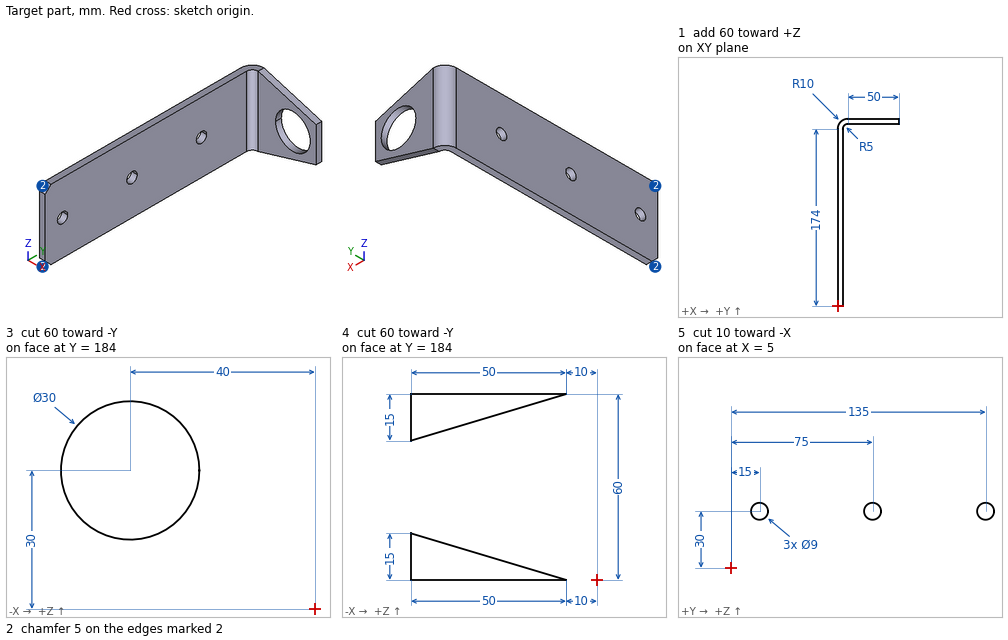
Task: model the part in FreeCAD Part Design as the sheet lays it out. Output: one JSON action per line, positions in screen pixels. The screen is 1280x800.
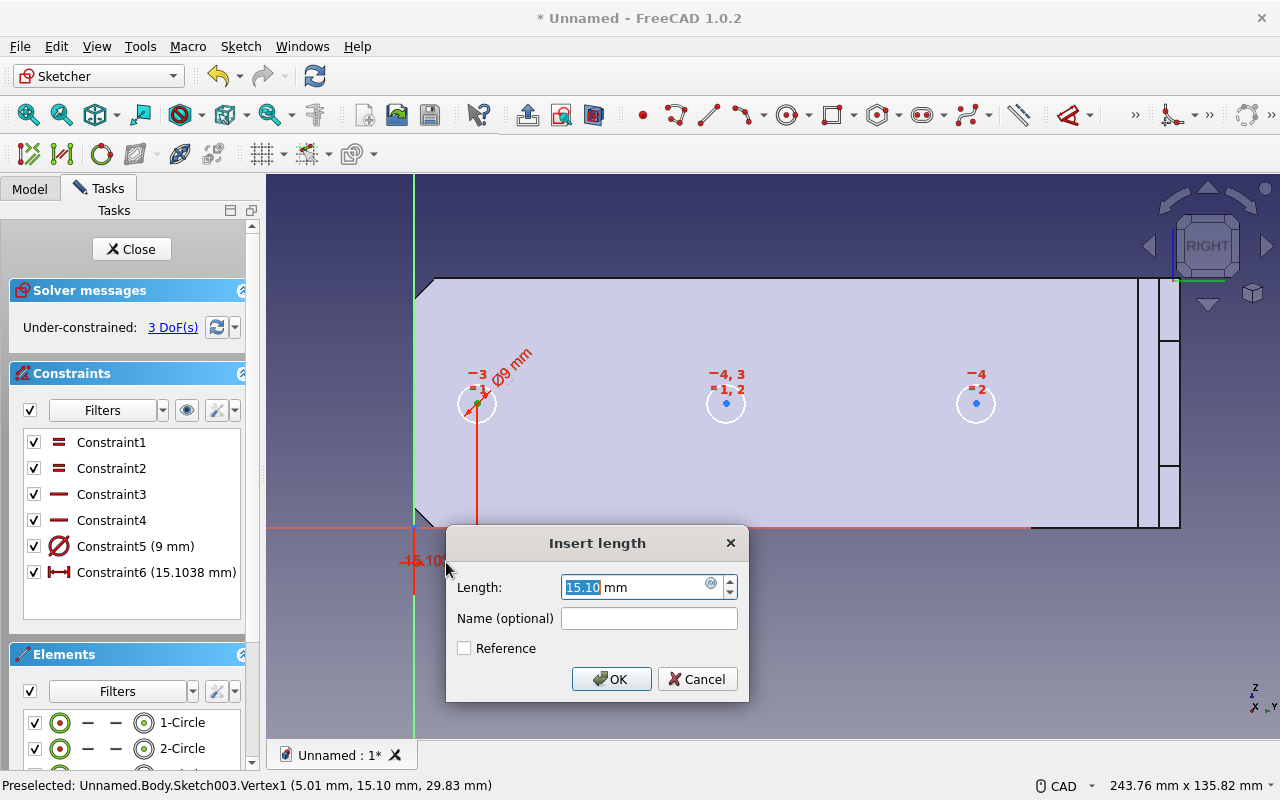
{"action": "type", "text": "15"}
{"action": "key", "text": "Return"}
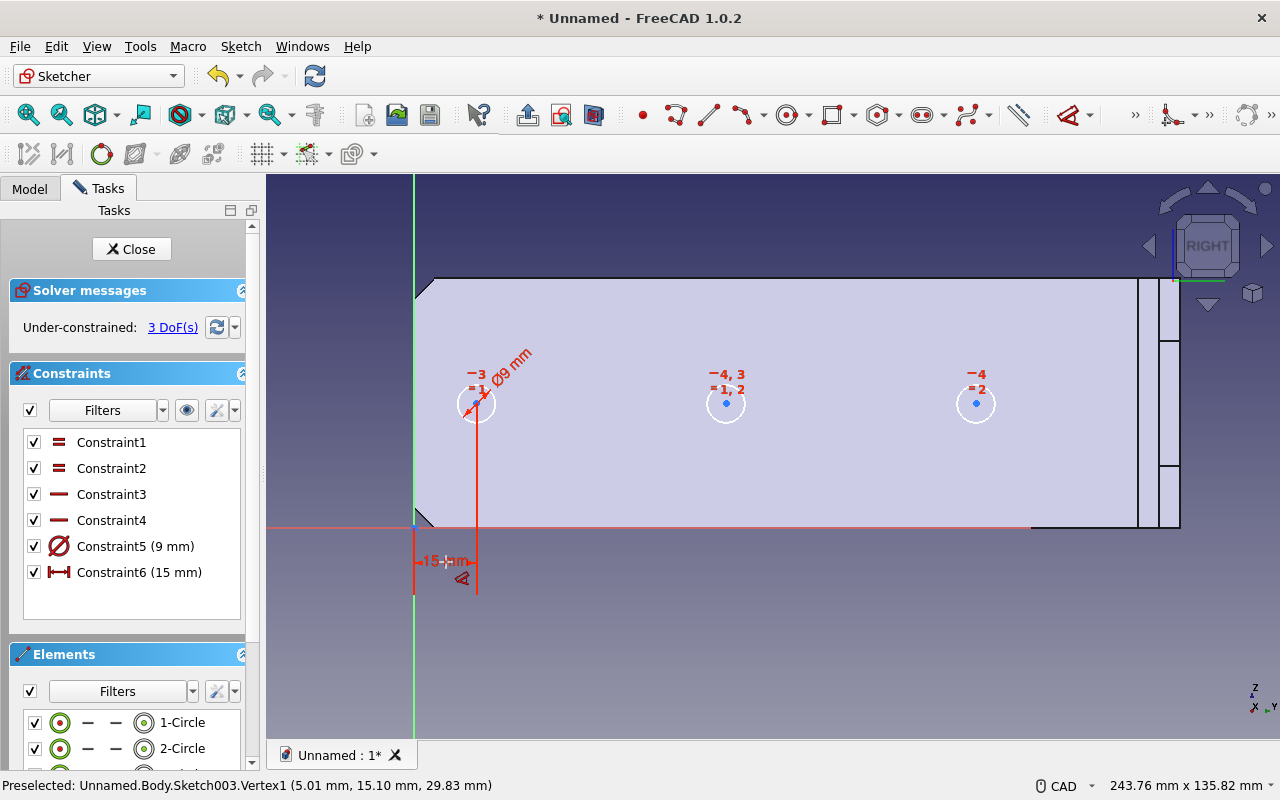
{"action": "left_click", "coordinate": [477, 404]}
{"action": "left_click", "coordinate": [380, 466]}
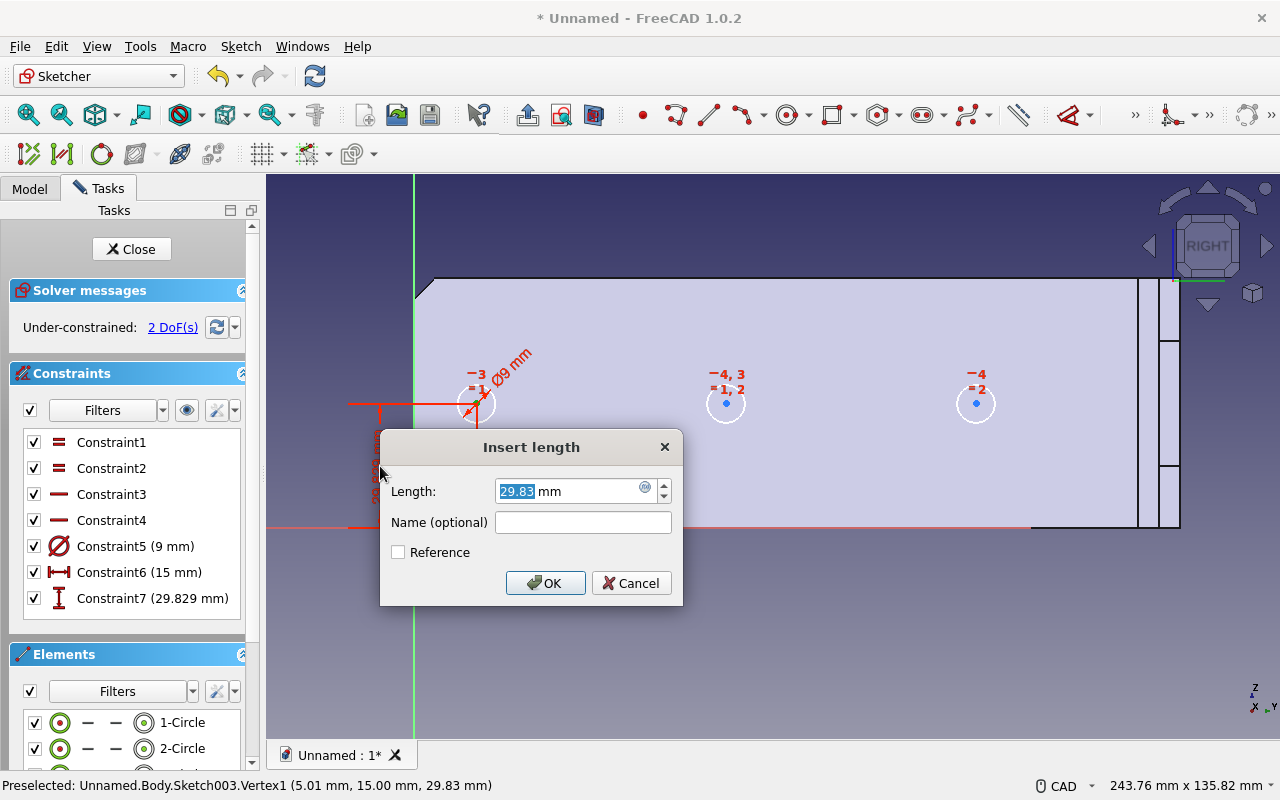
{"action": "type", "text": "30"}
{"action": "key", "text": "Return"}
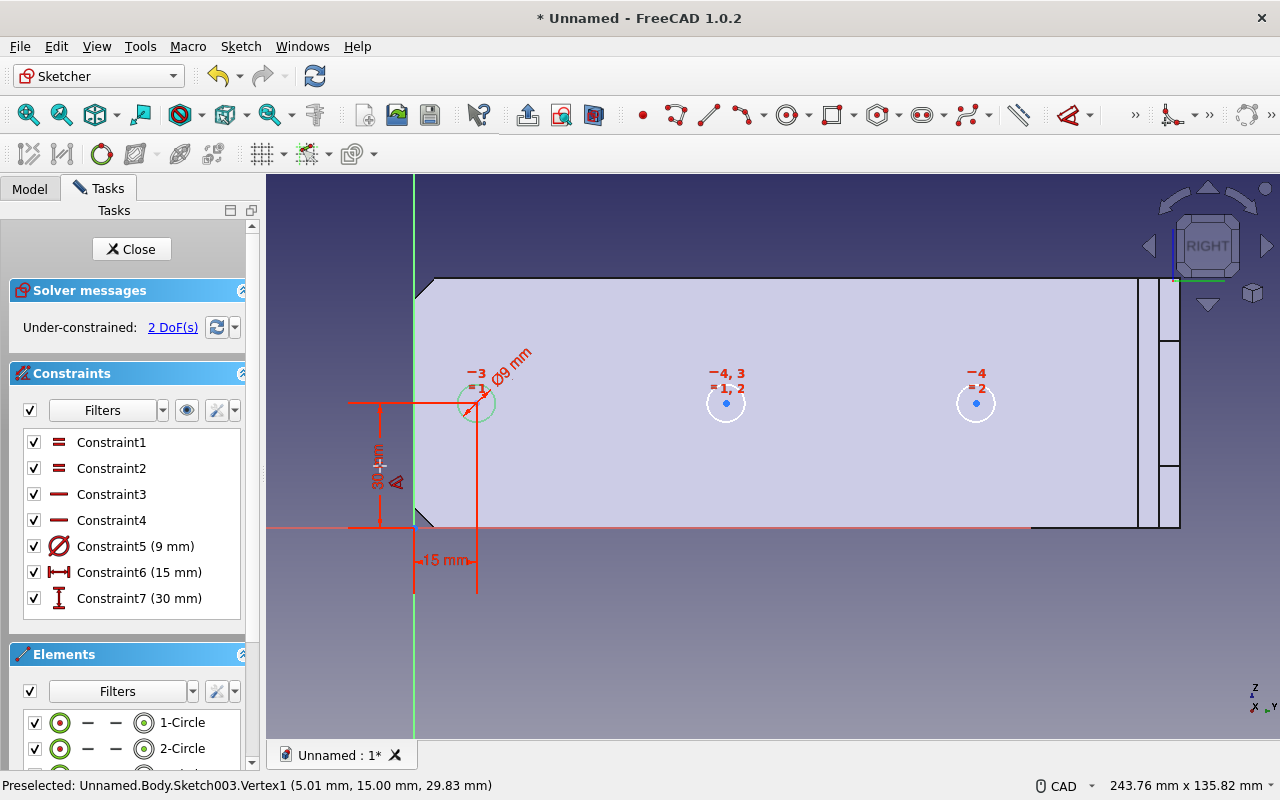
{"action": "left_click", "coordinate": [726, 403]}
{"action": "left_click", "coordinate": [570, 562]}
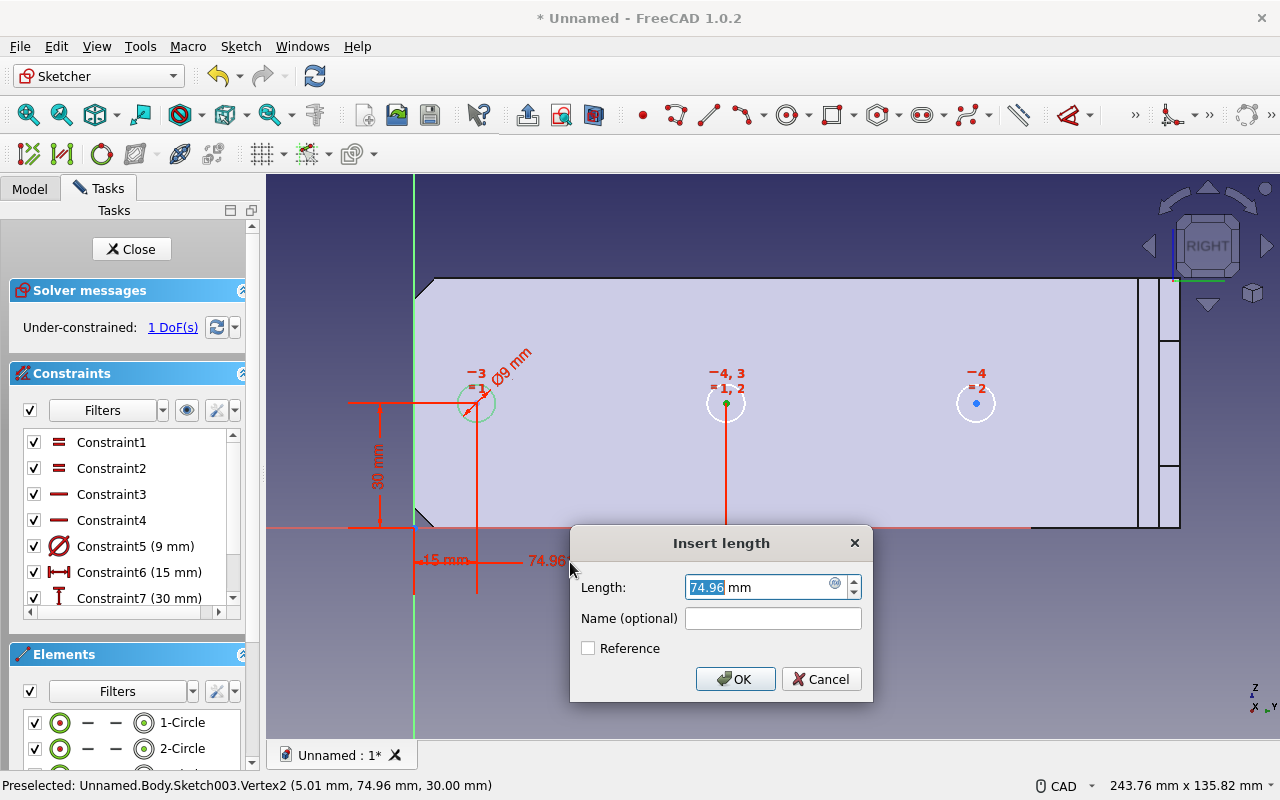
{"action": "type", "text": "75"}
{"action": "key", "text": "Return"}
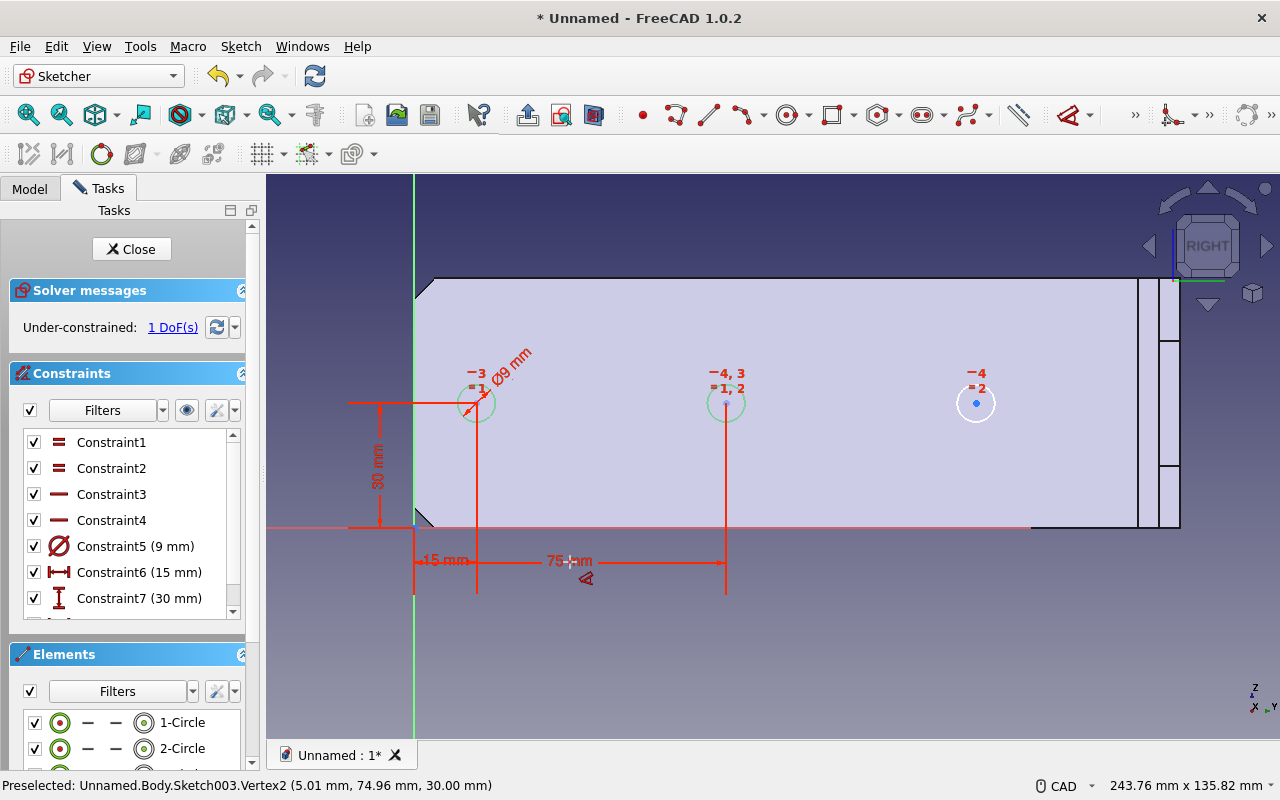
{"action": "left_click", "coordinate": [976, 403]}
{"action": "left_click", "coordinate": [695, 562]}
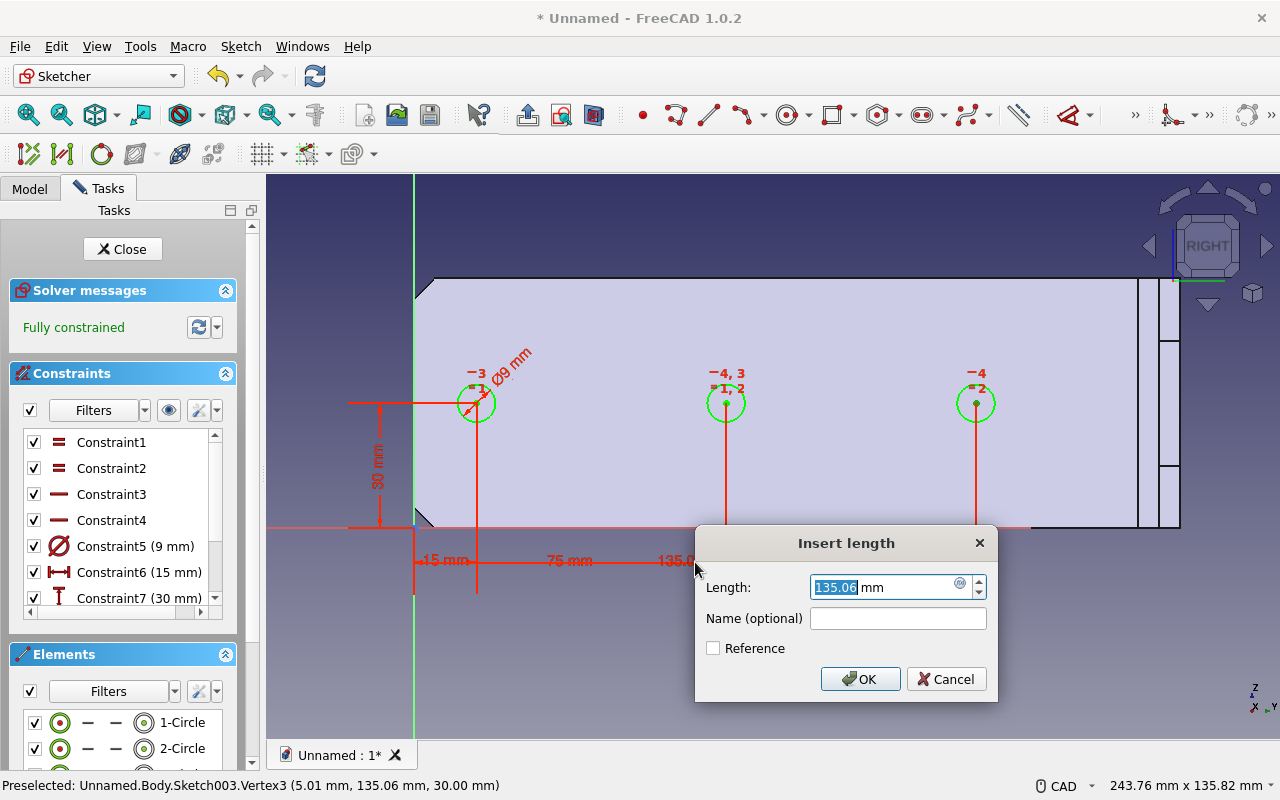
{"action": "type", "text": "135"}
{"action": "key", "text": "Return"}
{"action": "key", "text": "Escape"}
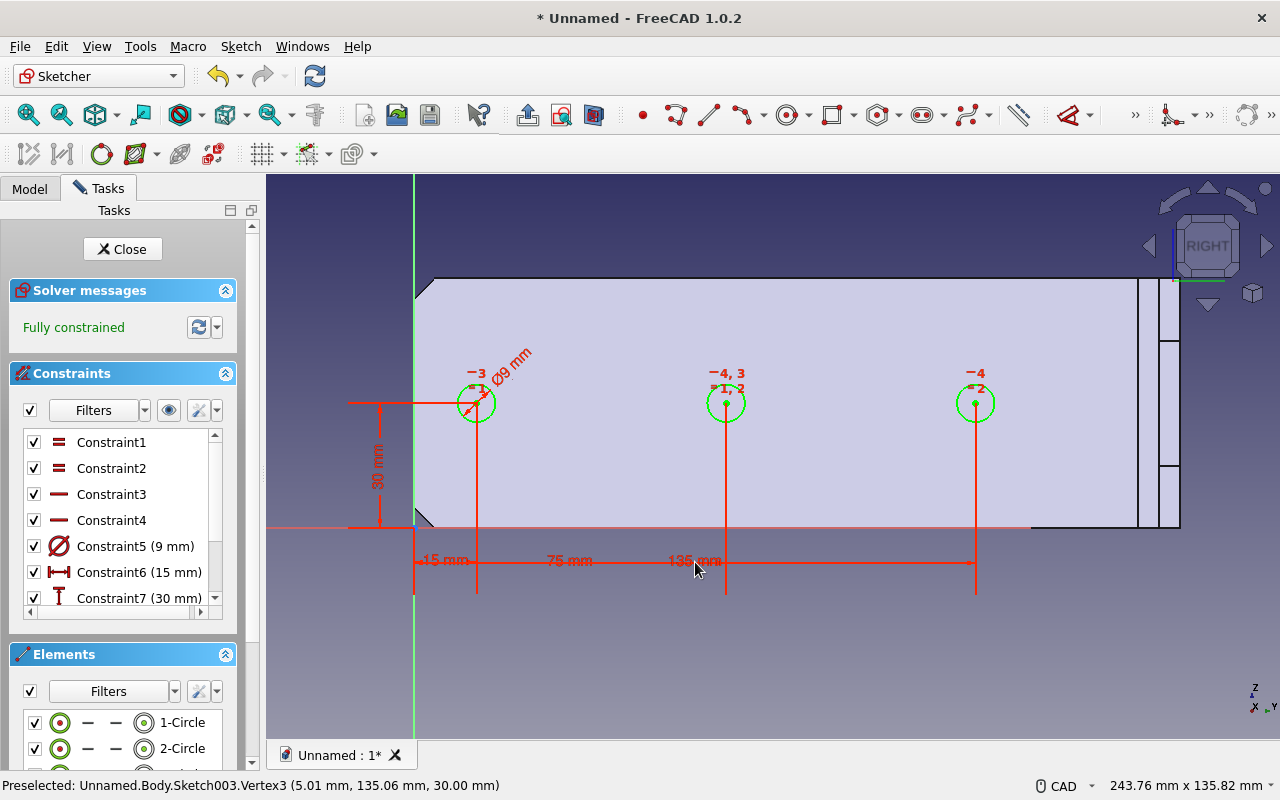
{"action": "left_click", "coordinate": [123, 249]}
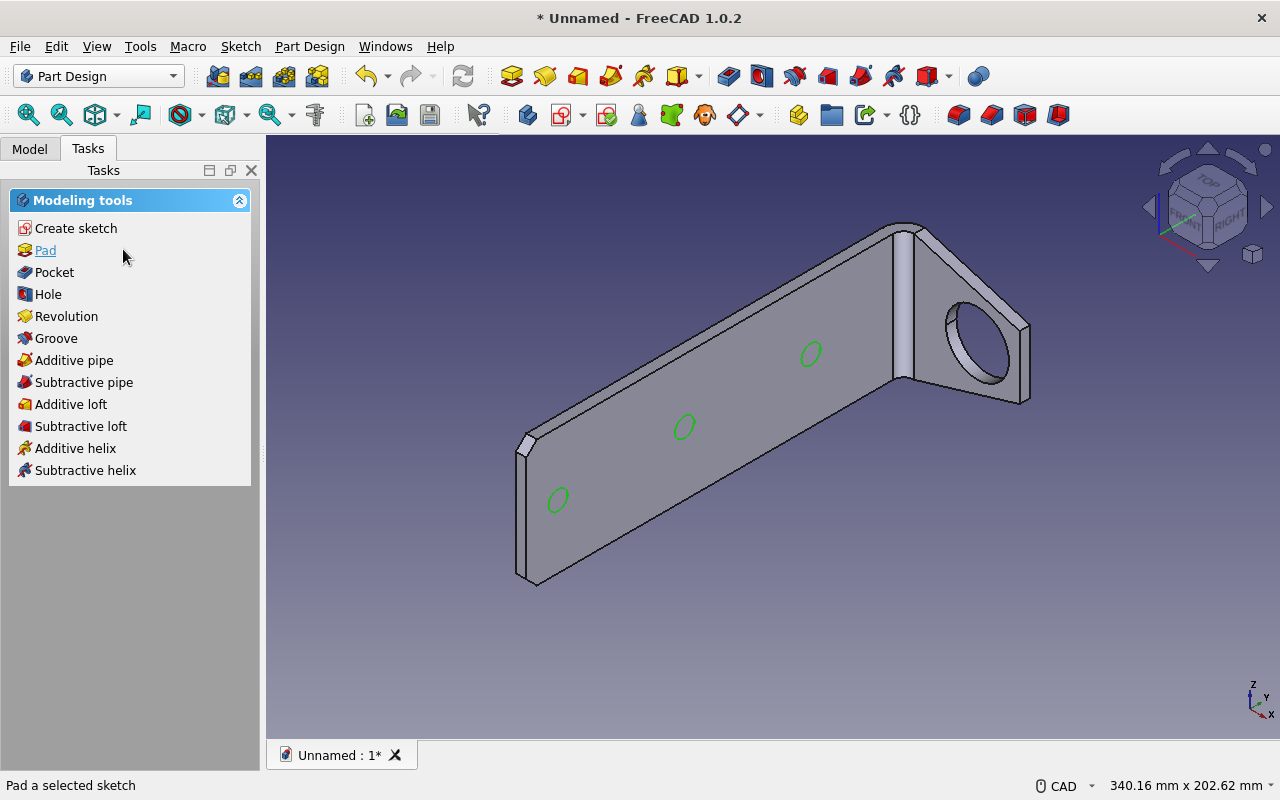
{"action": "left_click", "coordinate": [729, 76]}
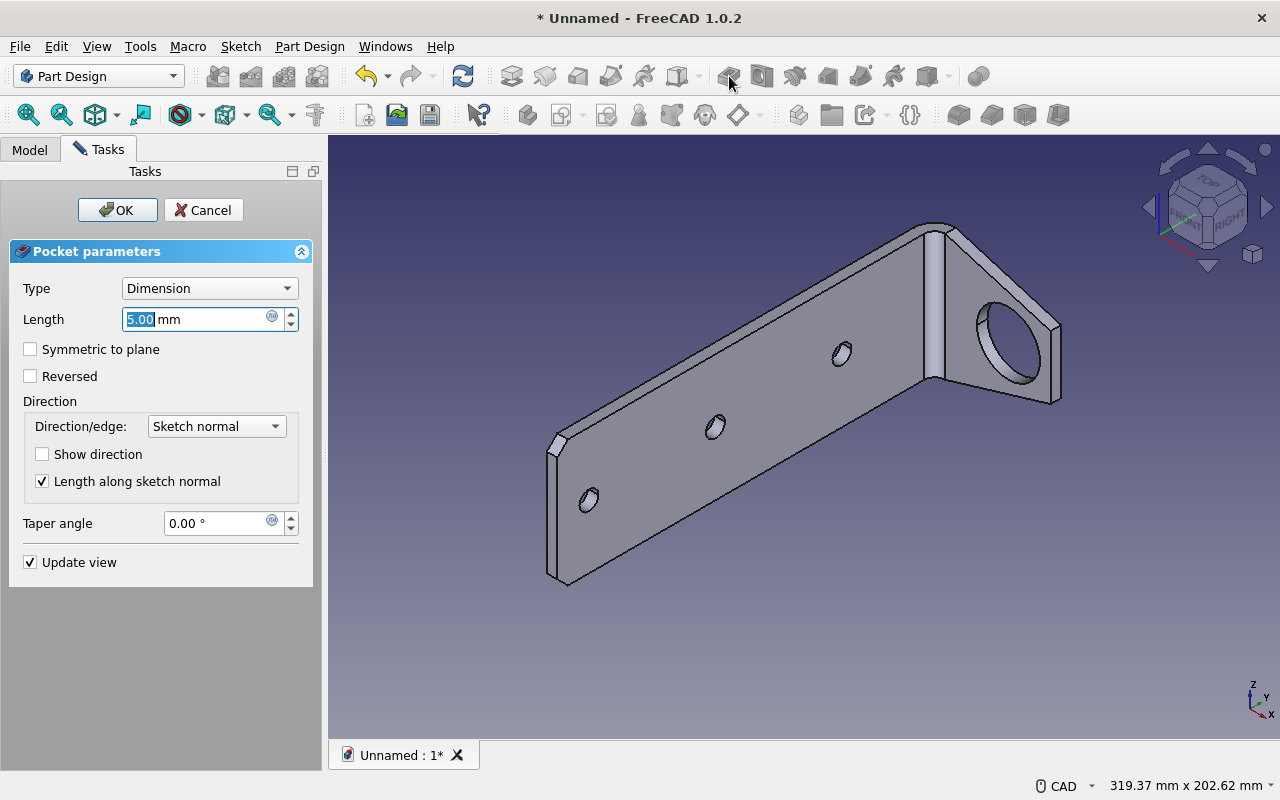
{"action": "type", "text": "10"}
{"action": "key", "text": "Tab"}